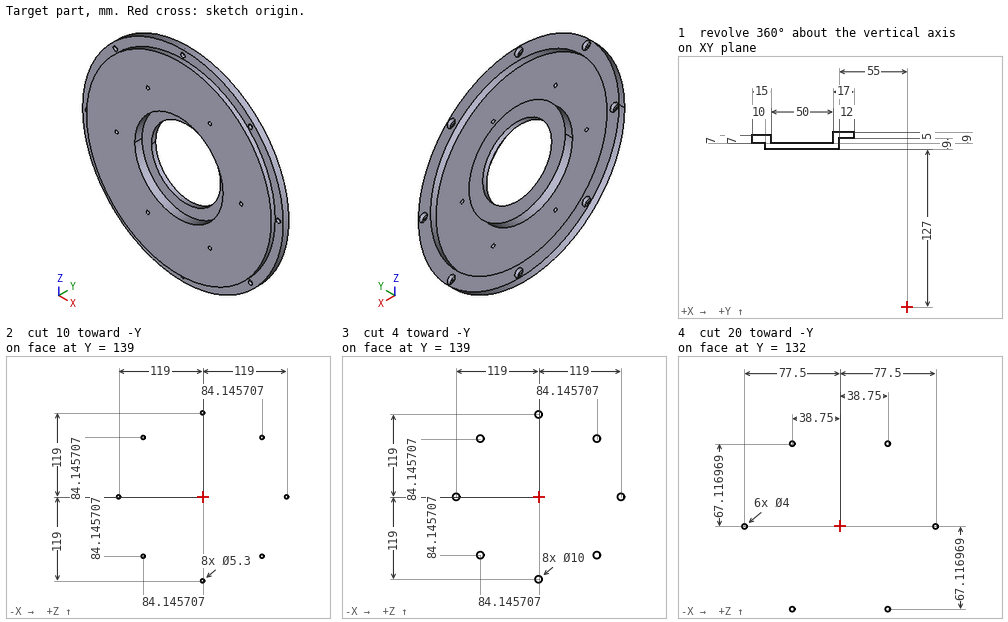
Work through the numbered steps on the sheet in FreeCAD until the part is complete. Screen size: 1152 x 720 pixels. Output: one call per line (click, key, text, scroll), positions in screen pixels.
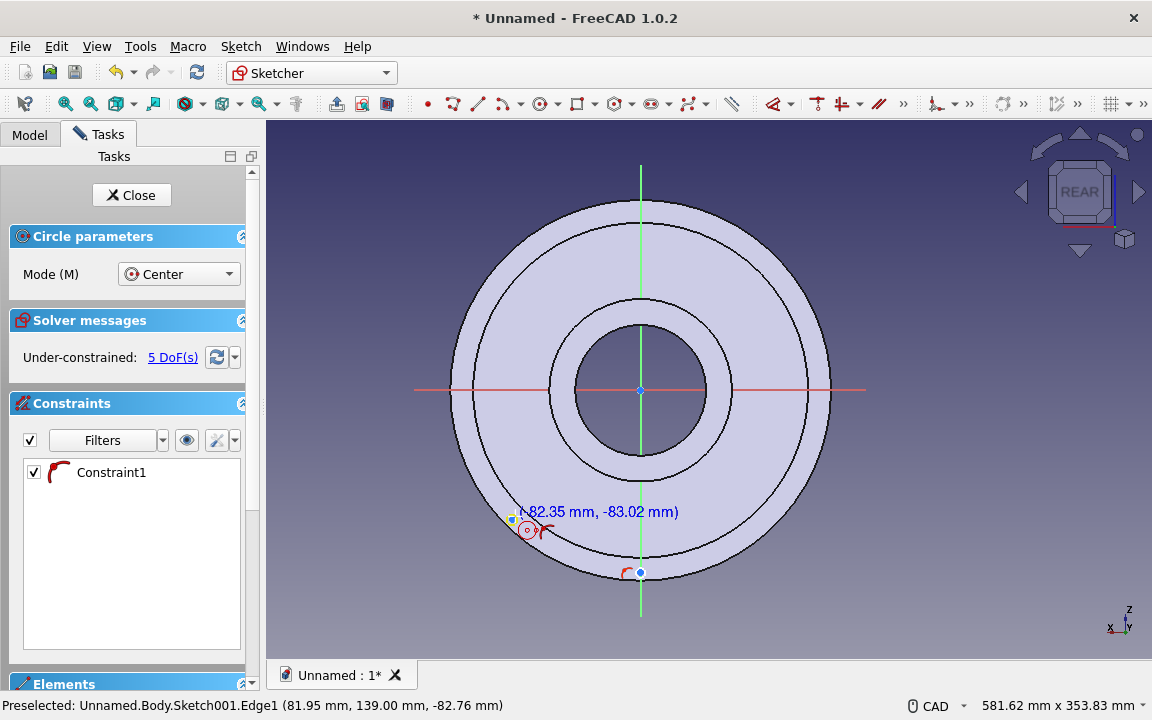
scroll(459, 390, up, 9)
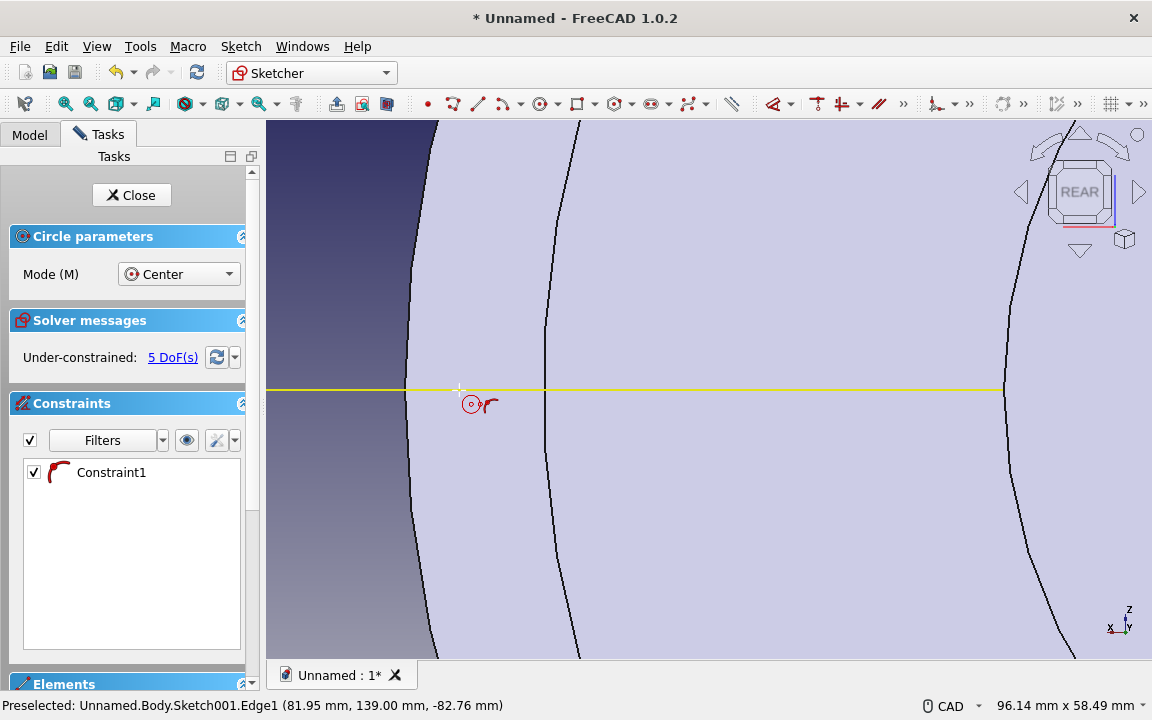
scroll(459, 389, down, 9)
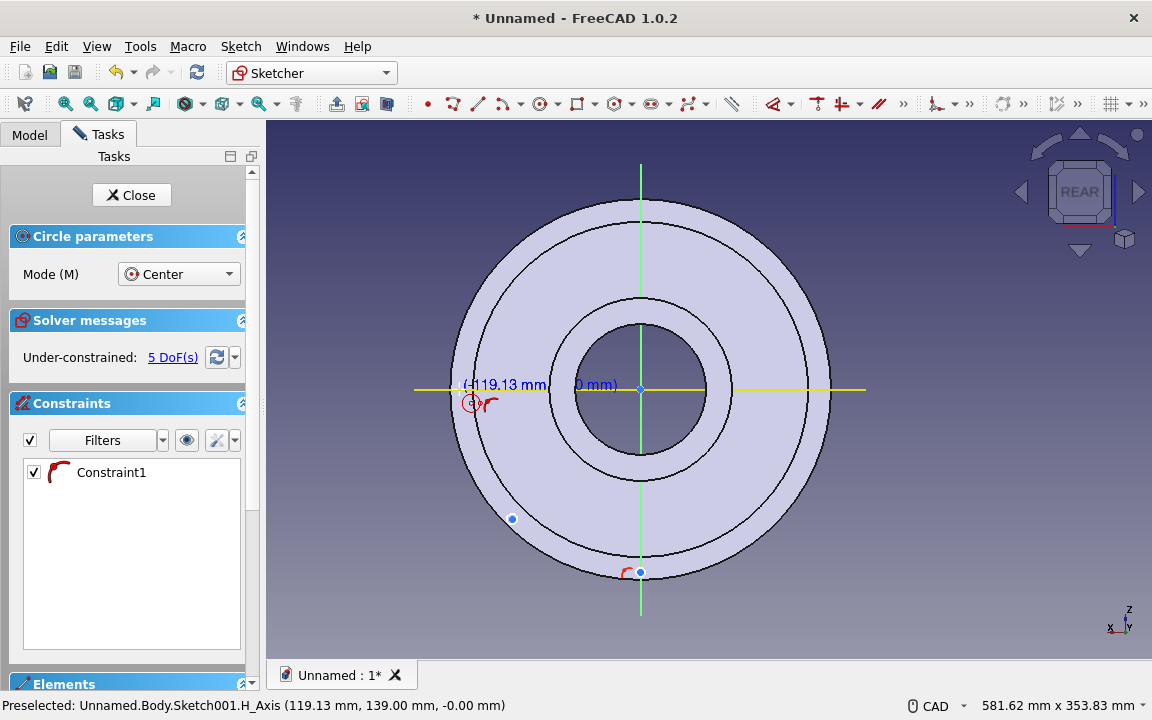
click(459, 390)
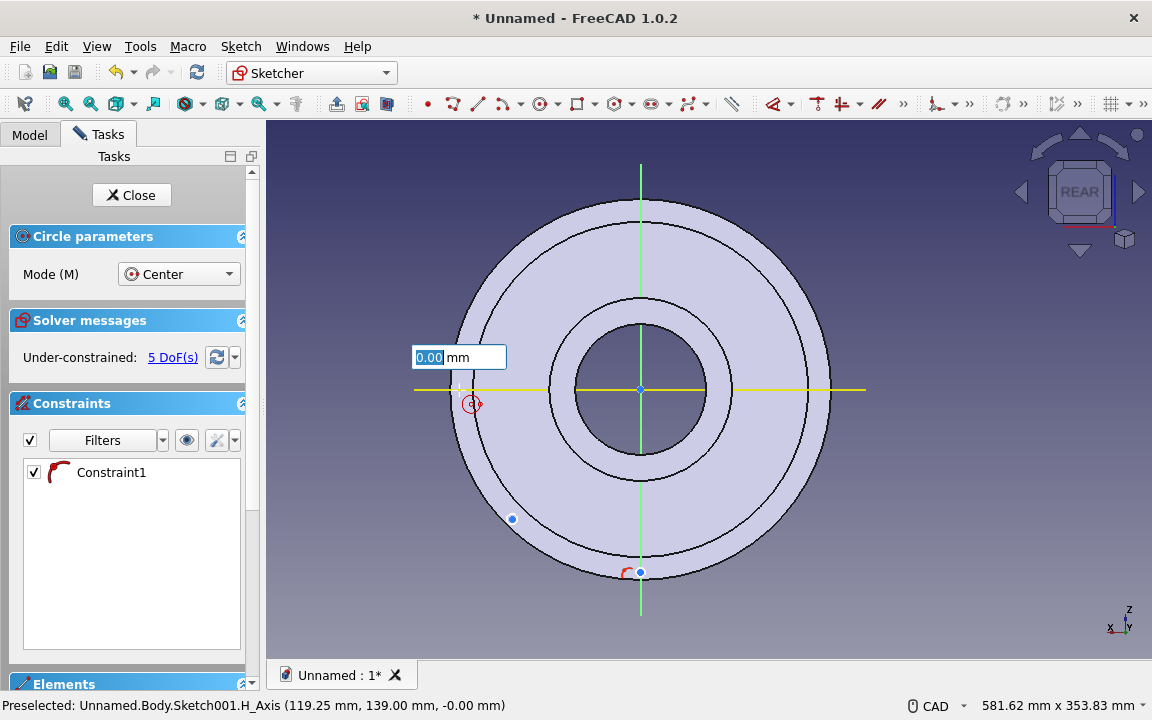
scroll(458, 393, up, 8)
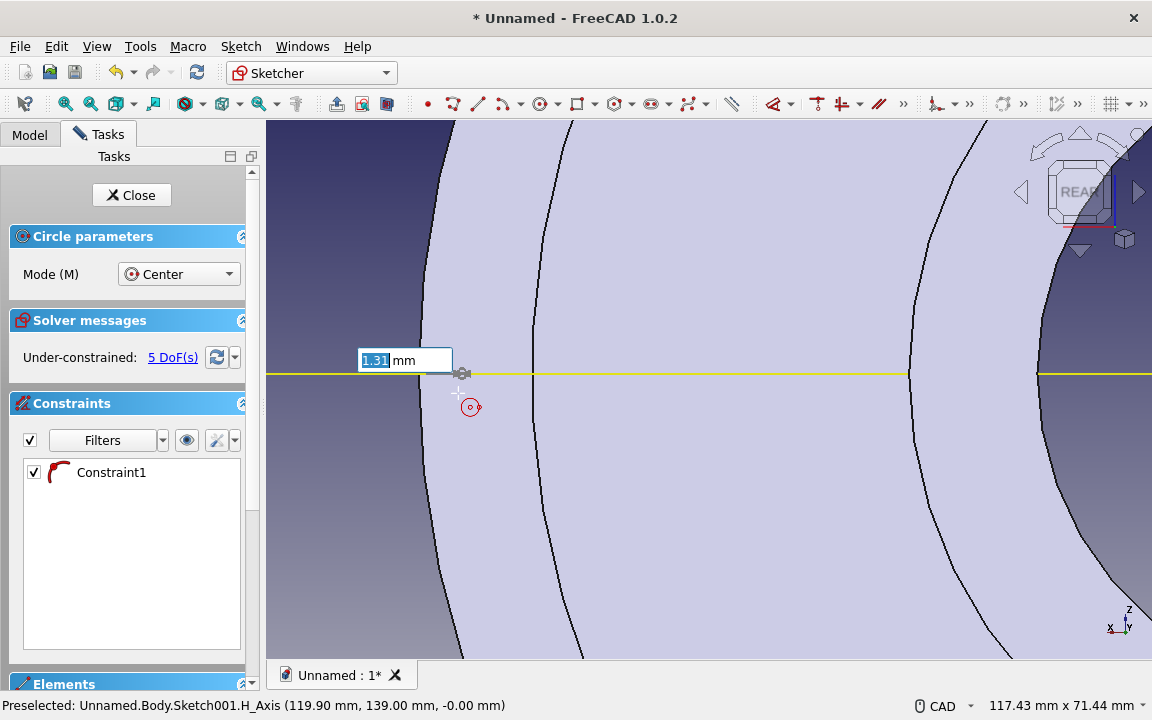
click(457, 392)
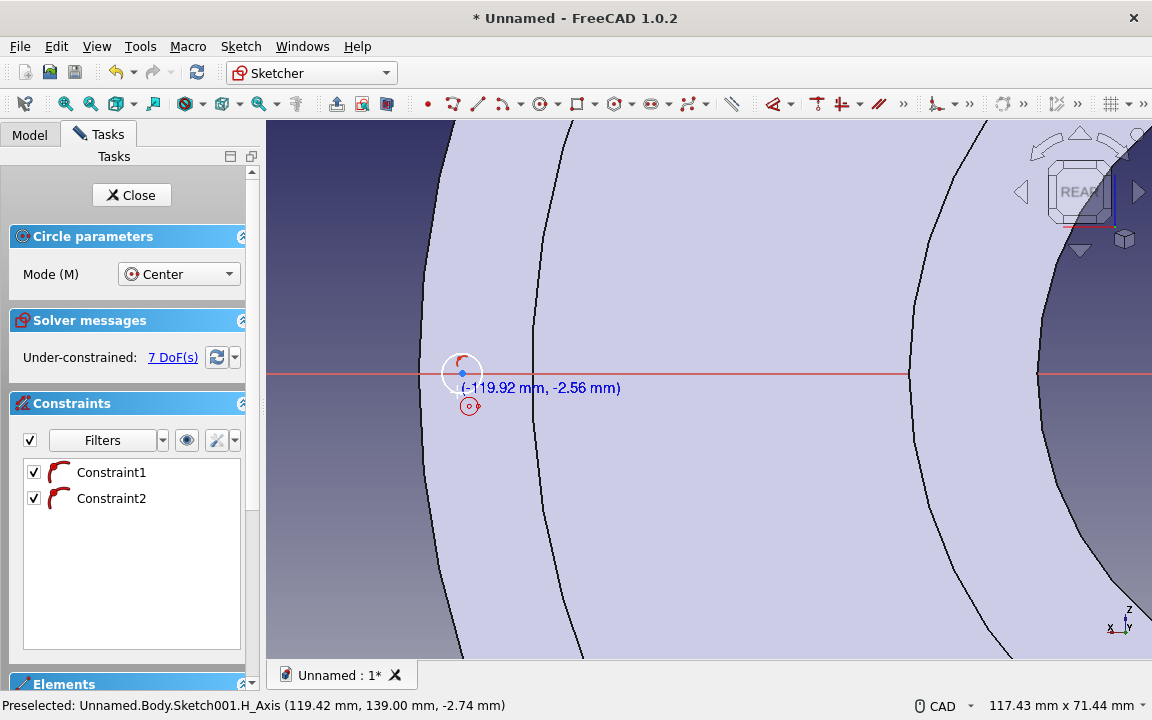
scroll(458, 394, down, 8)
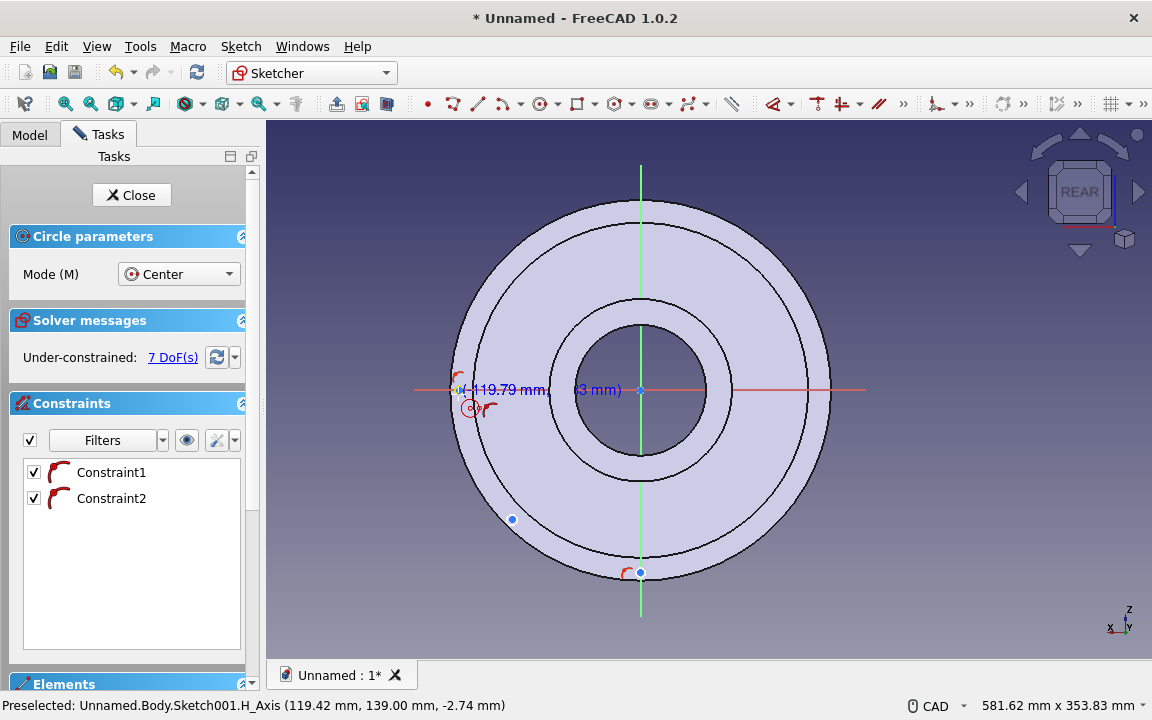
scroll(512, 262, up, 9)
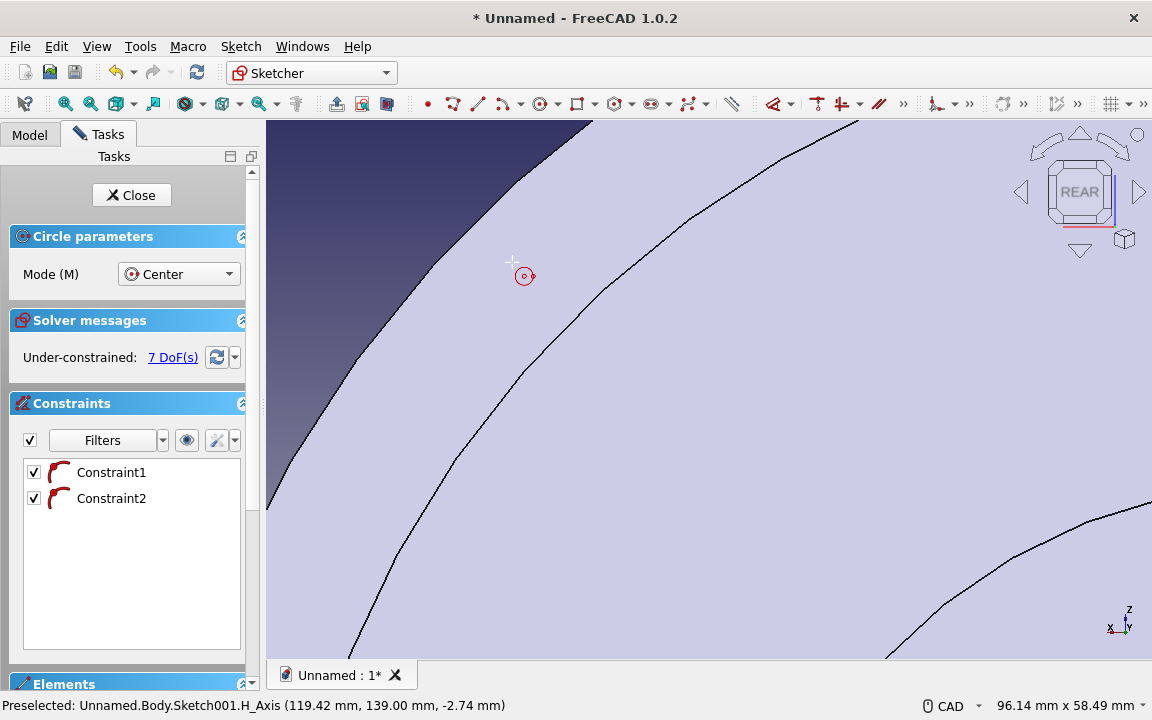
scroll(512, 261, down, 9)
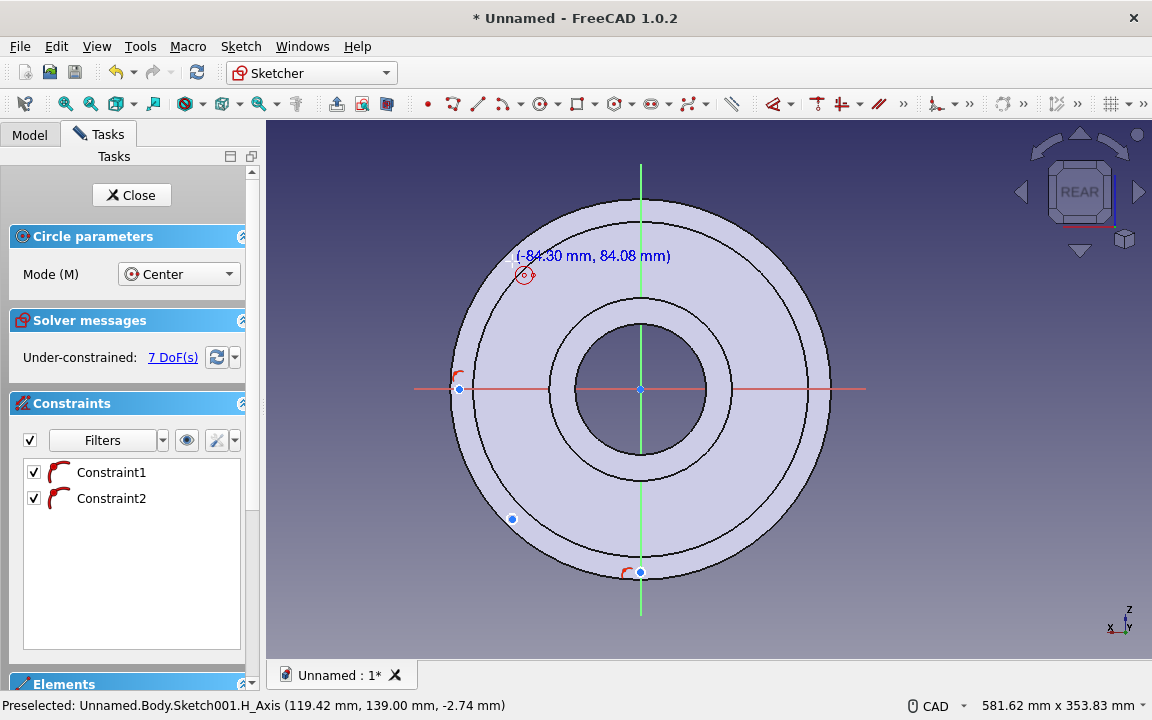
click(512, 261)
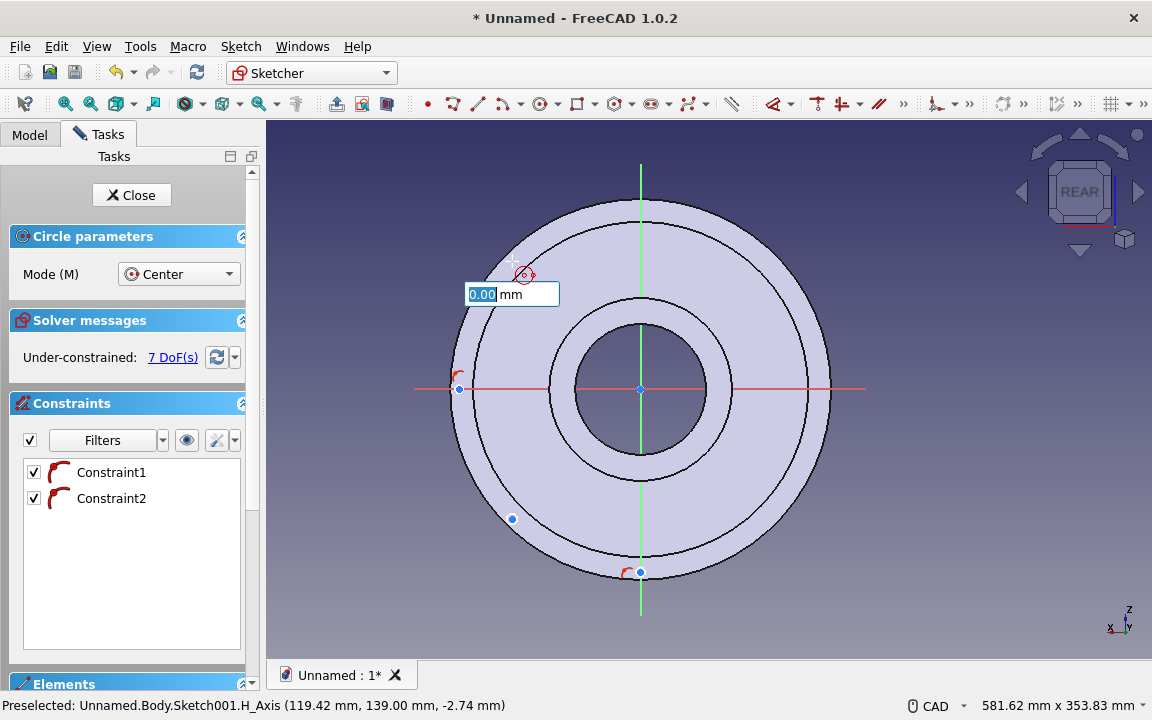
scroll(515, 258, up, 7)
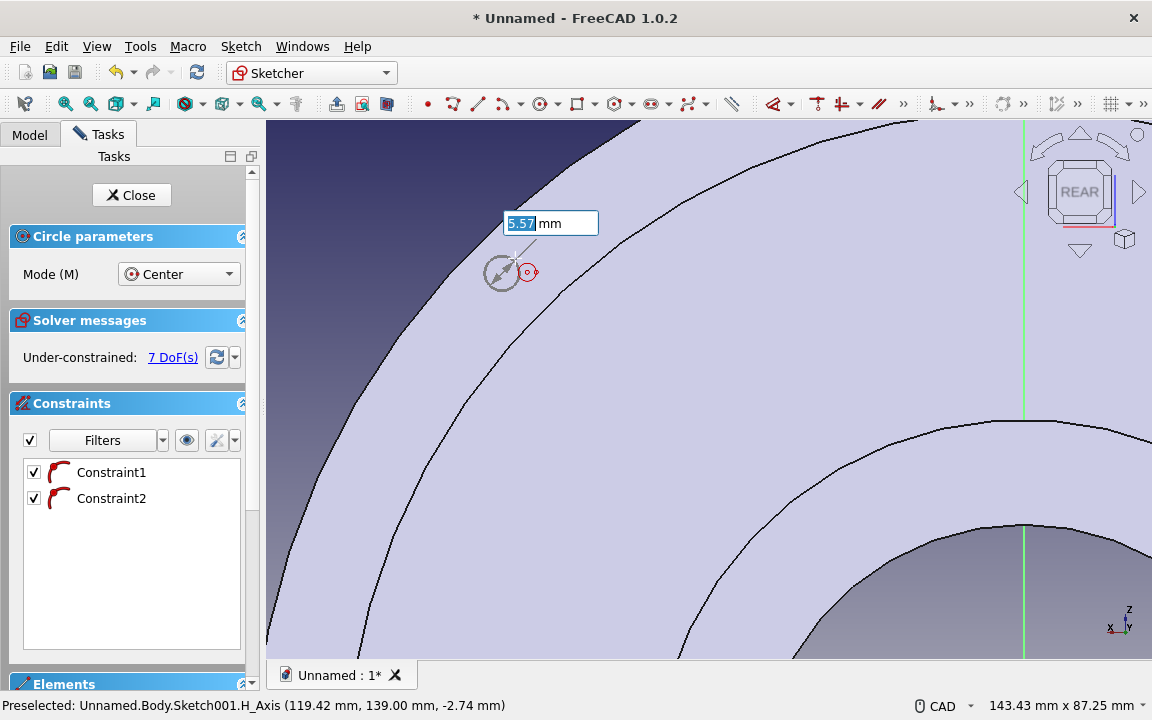
click(515, 259)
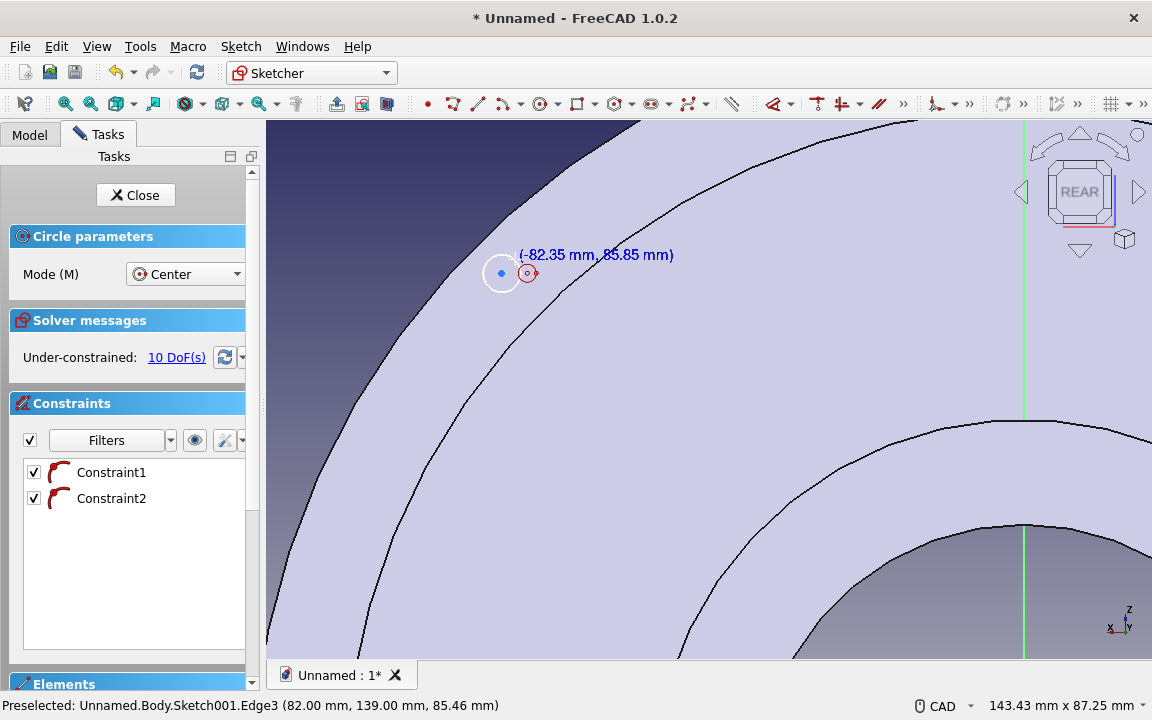
scroll(515, 258, down, 7)